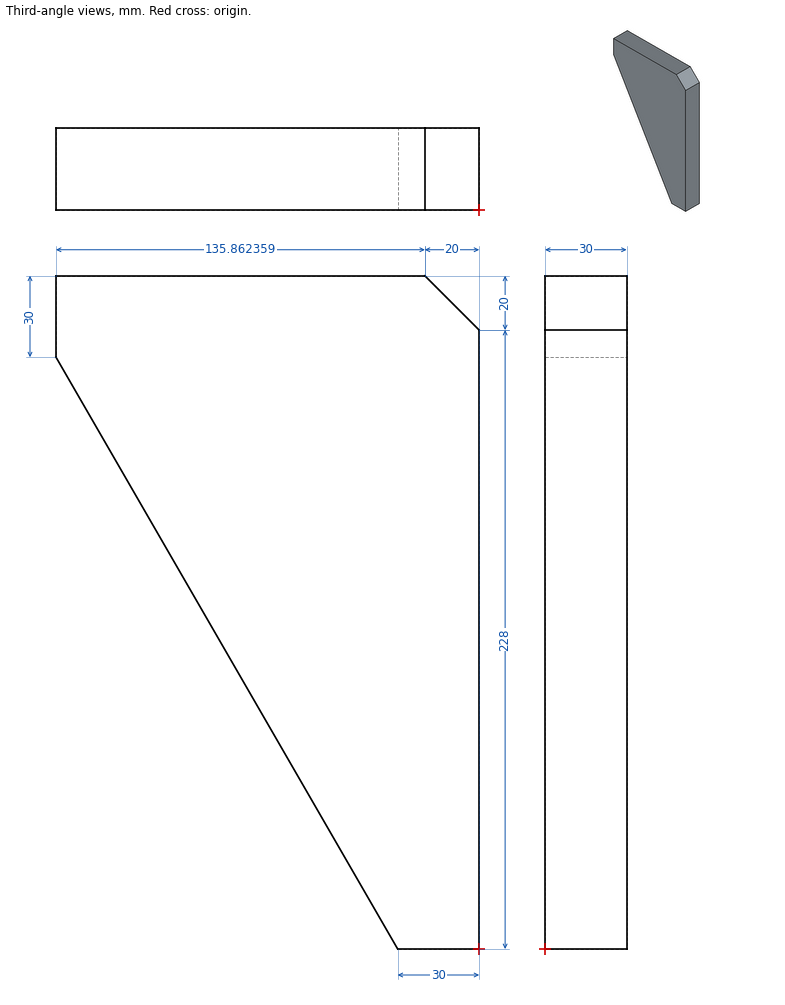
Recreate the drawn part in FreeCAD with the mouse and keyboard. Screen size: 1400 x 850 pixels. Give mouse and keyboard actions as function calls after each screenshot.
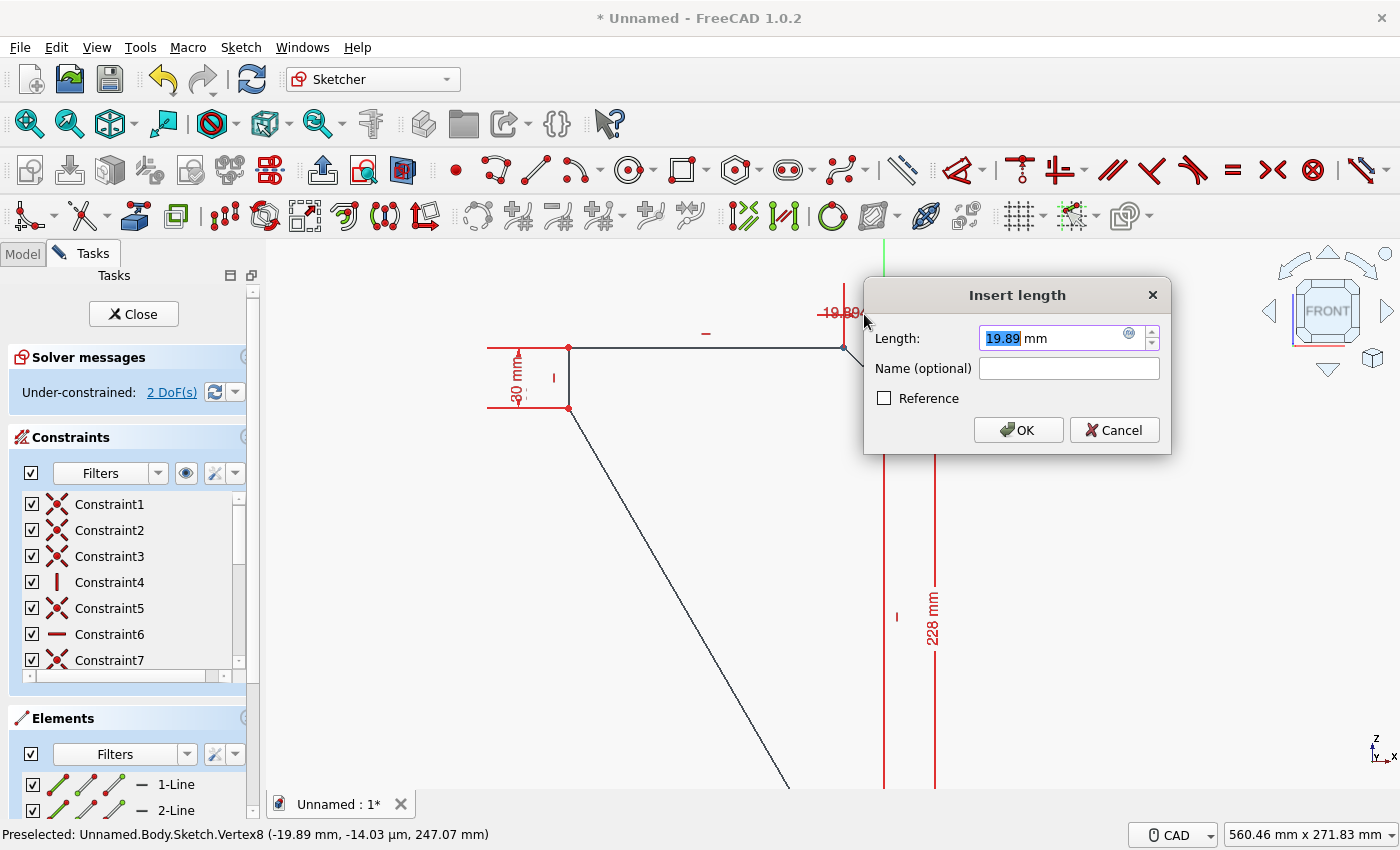
text(20)
key(Return)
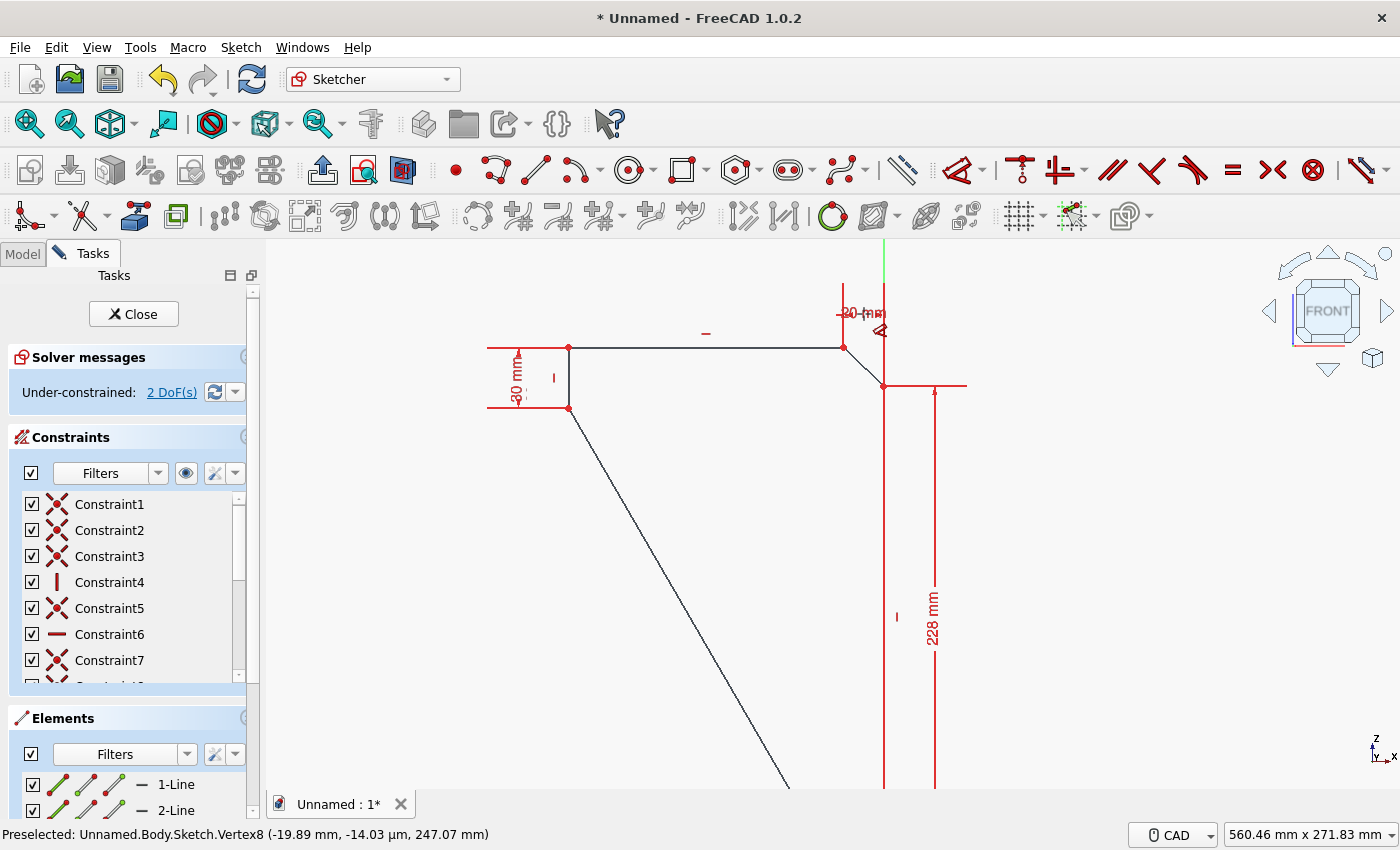
click(856, 359)
click(918, 367)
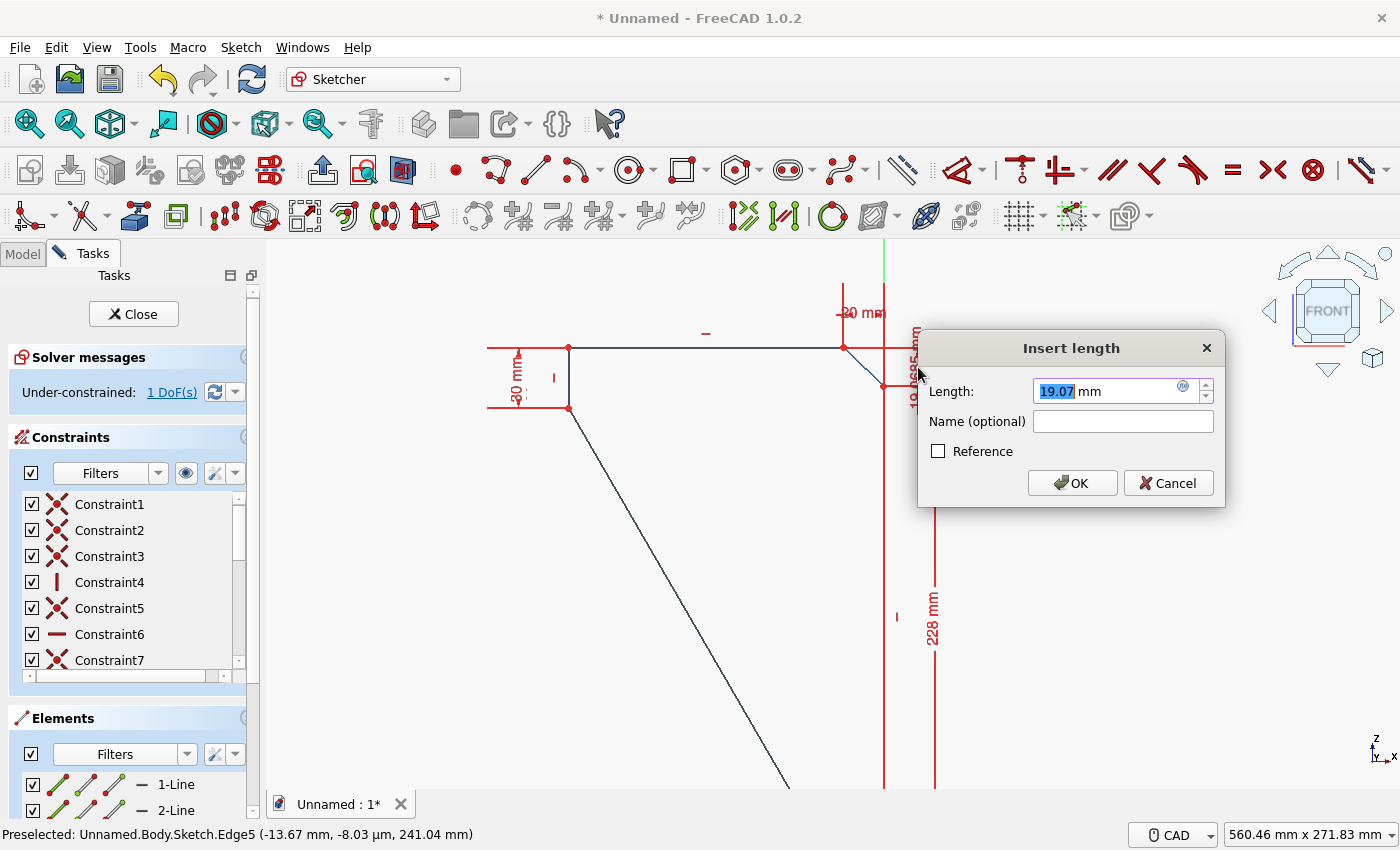
text(20)
key(Return)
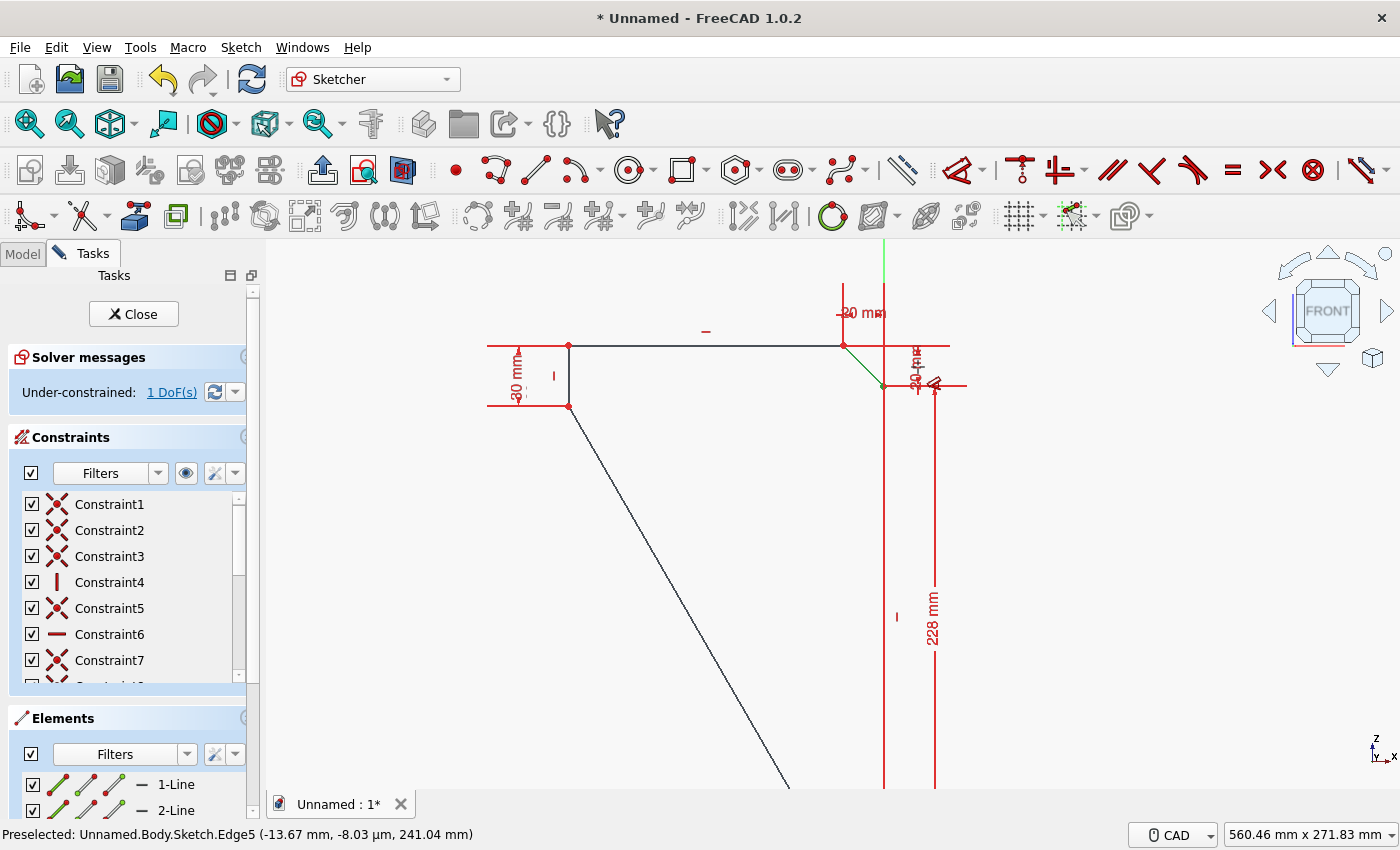
click(651, 346)
click(706, 312)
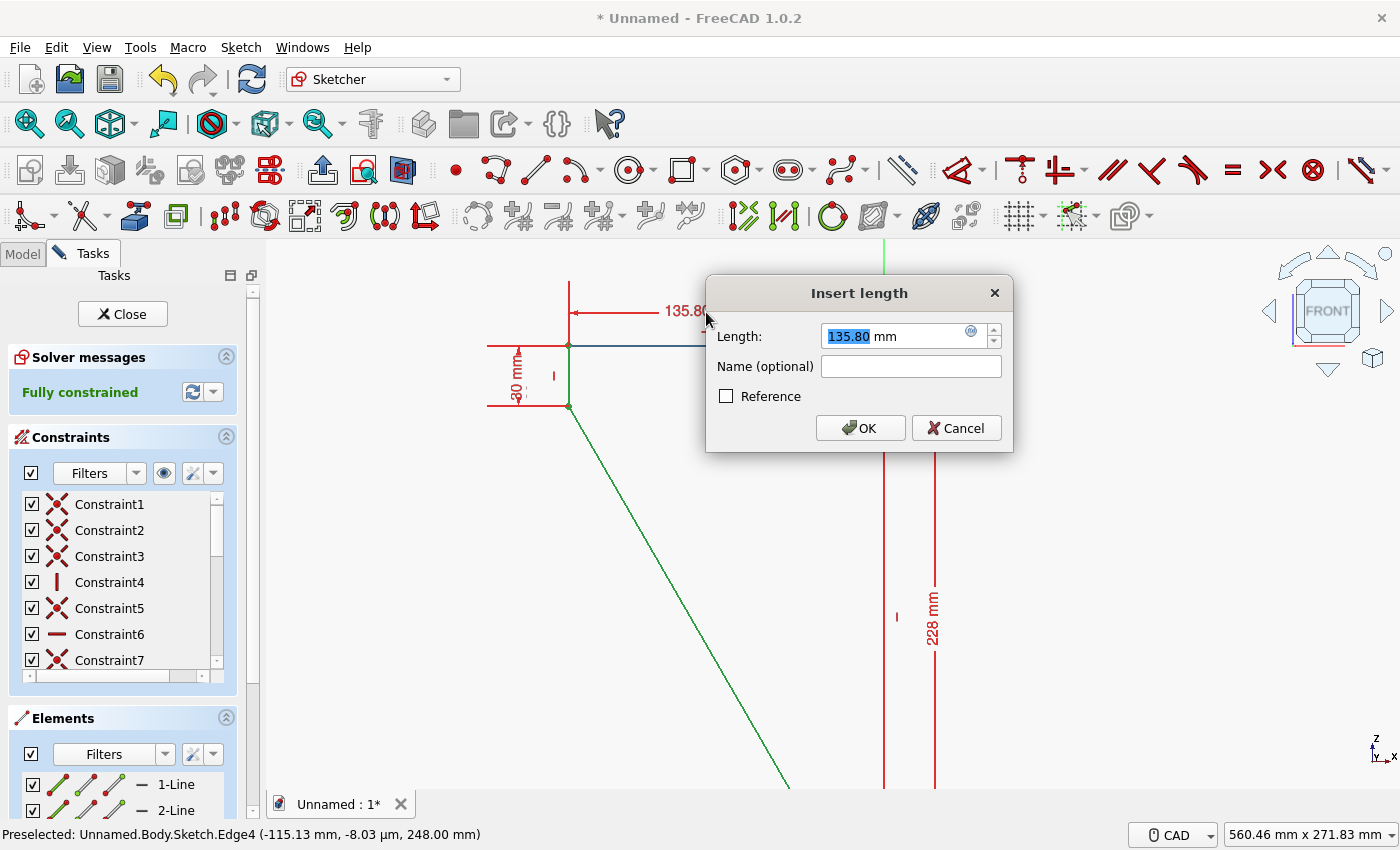
text(135.862359)
key(Return)
key(Escape)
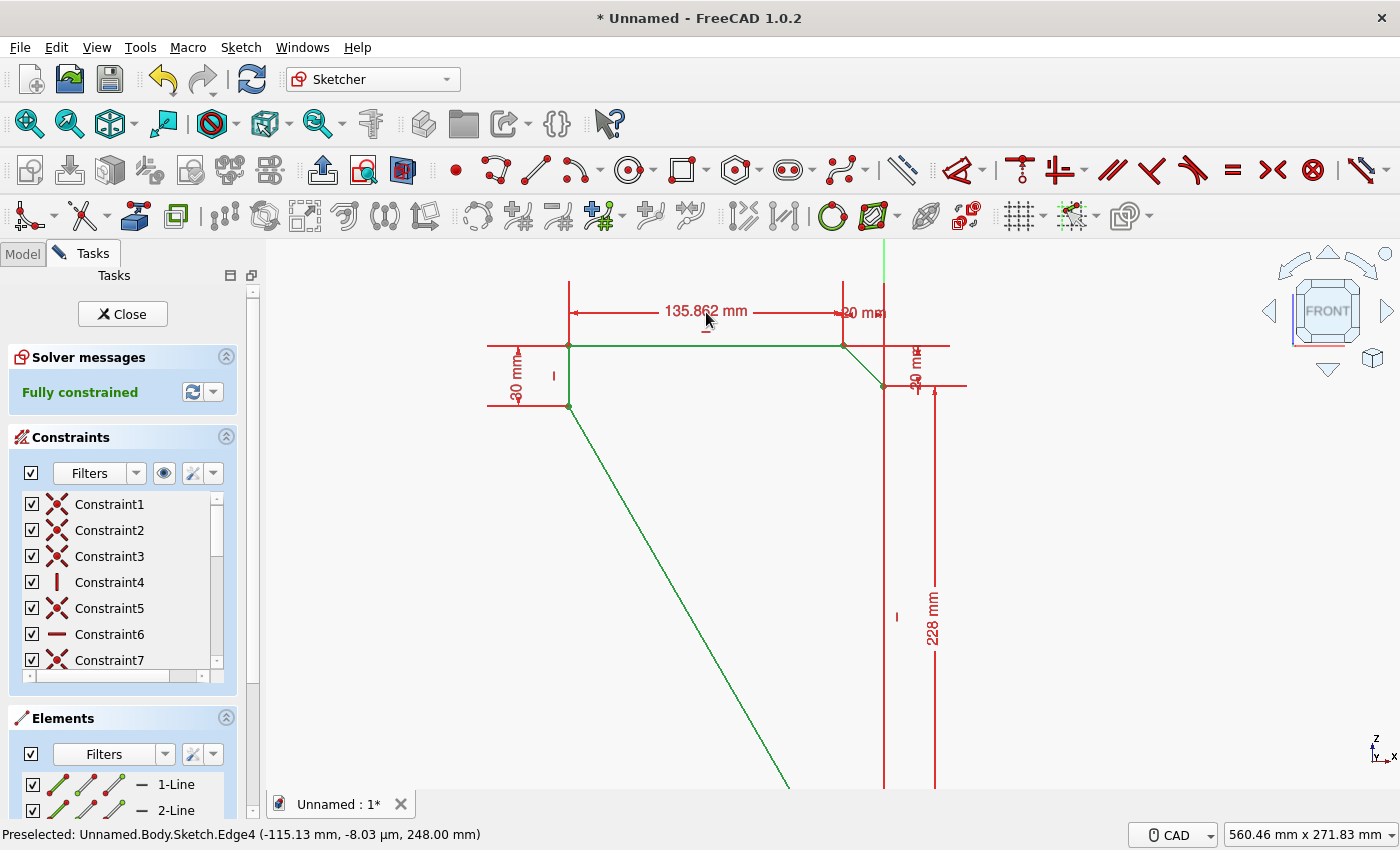
click(123, 314)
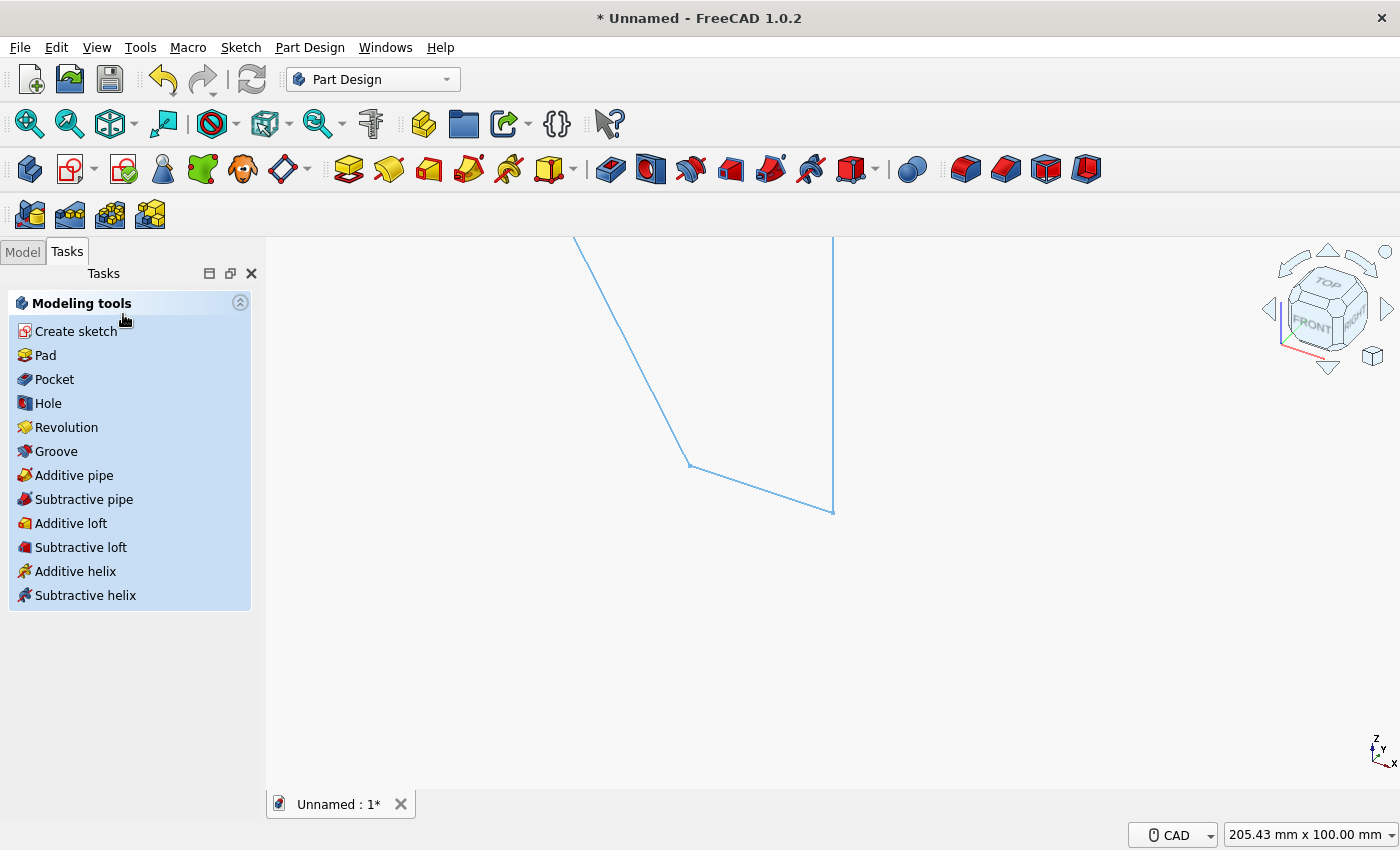
click(350, 170)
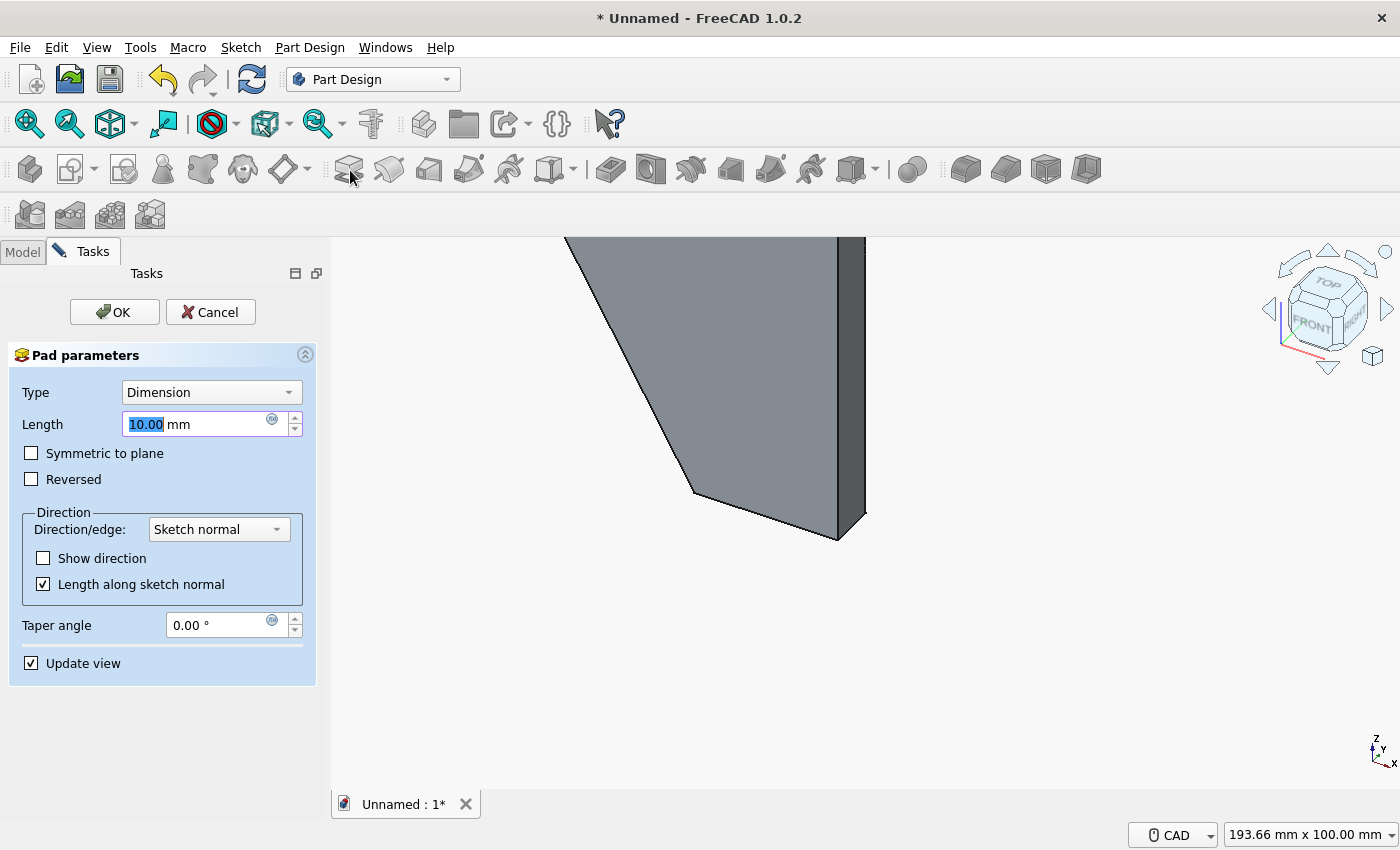
text(30)
key(Tab)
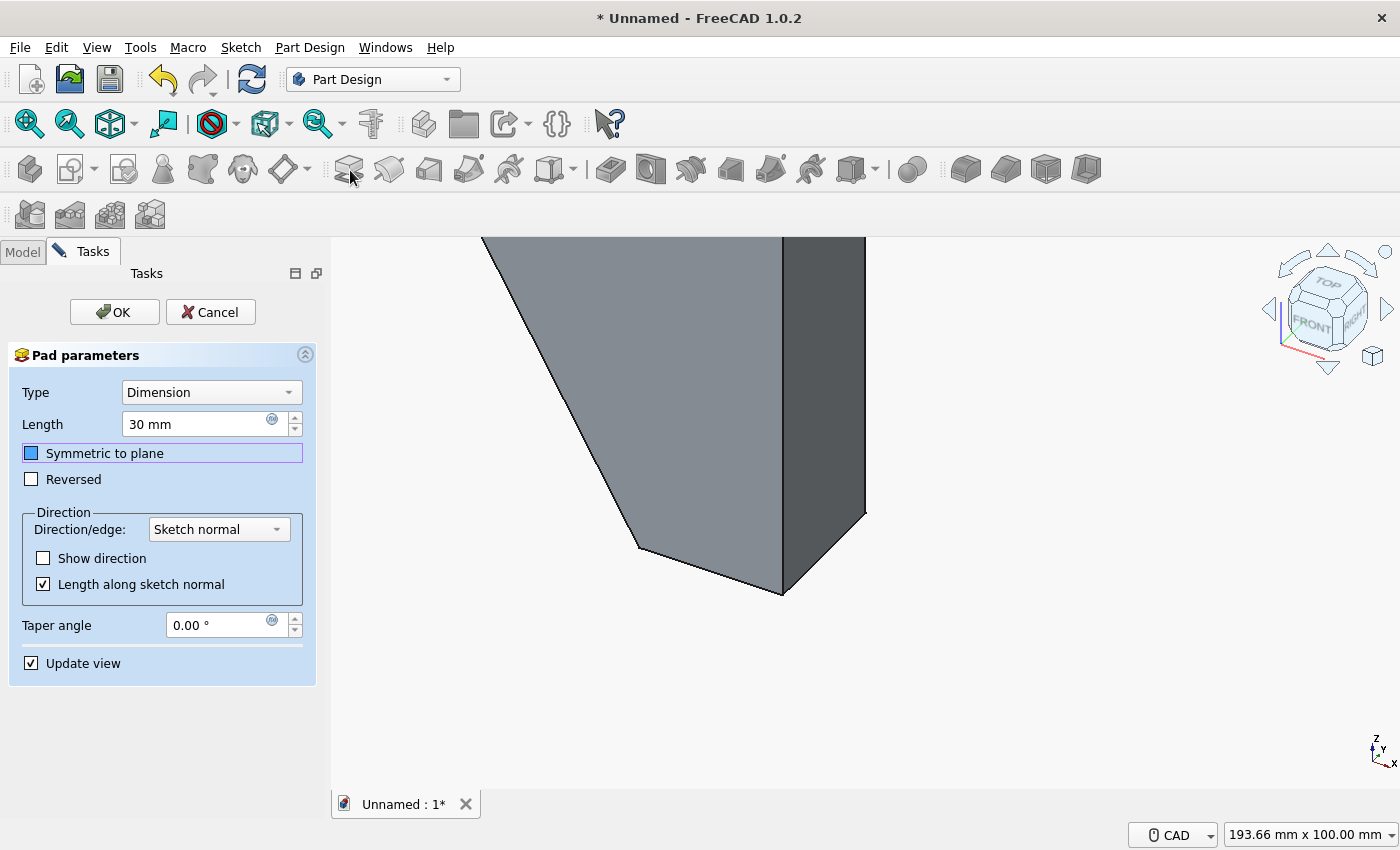
click(30, 479)